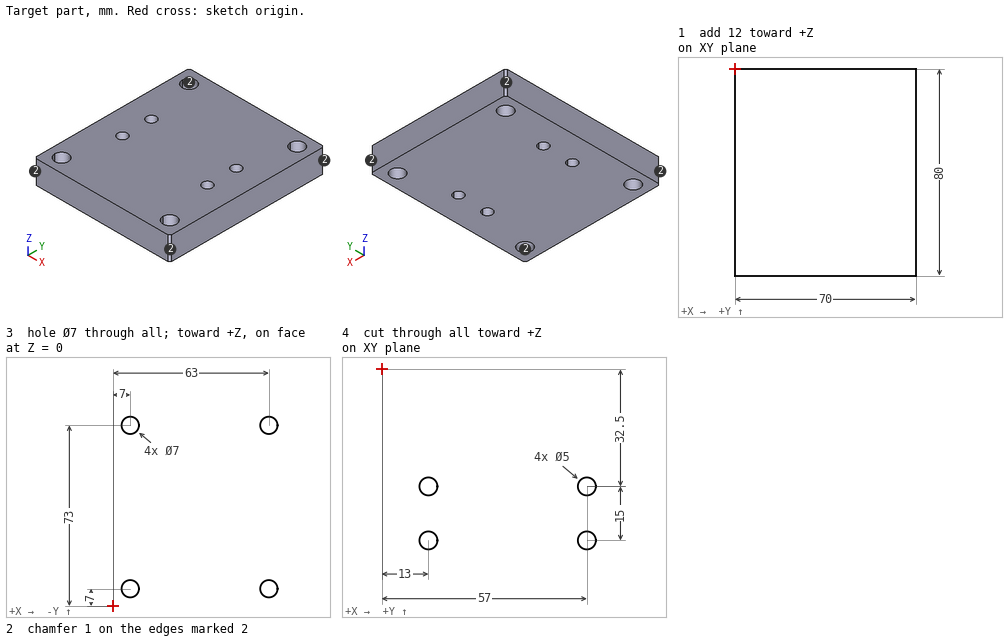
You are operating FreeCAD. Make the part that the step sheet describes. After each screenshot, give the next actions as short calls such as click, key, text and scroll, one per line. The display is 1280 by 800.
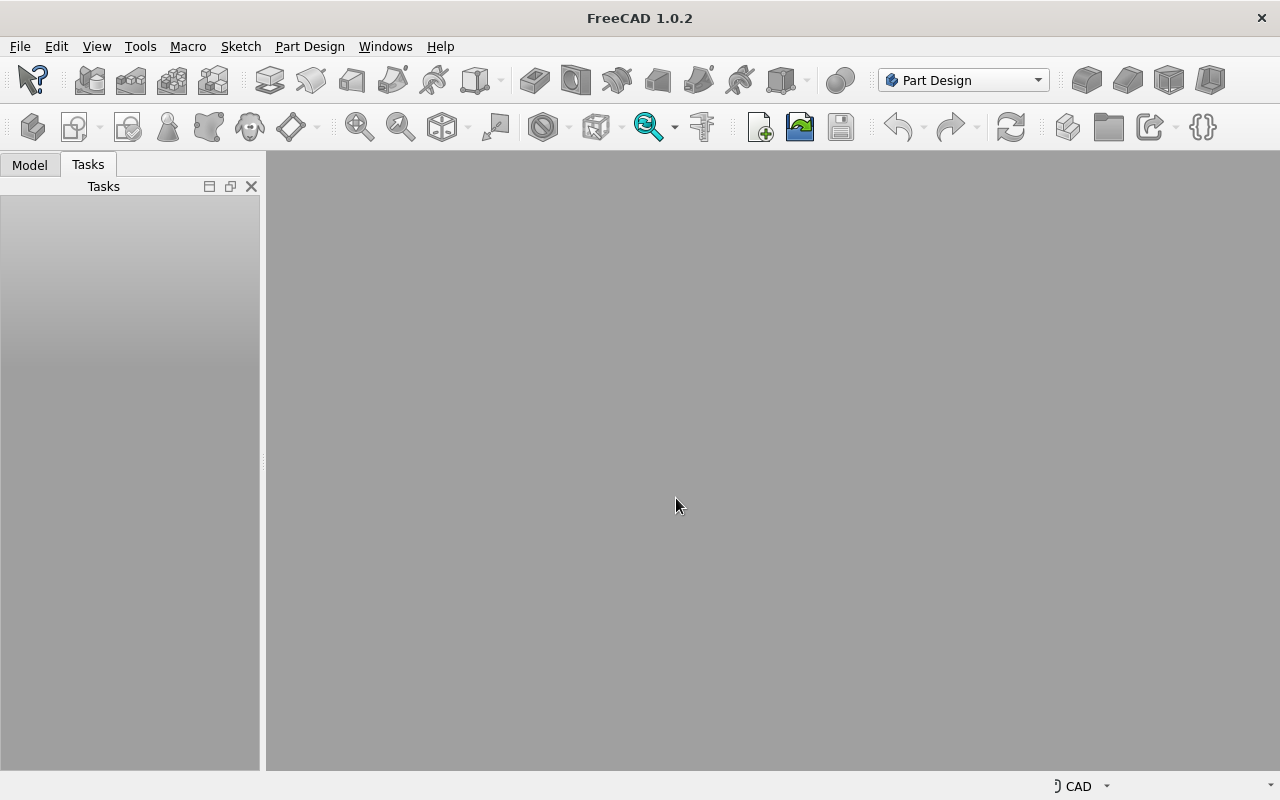
click(759, 128)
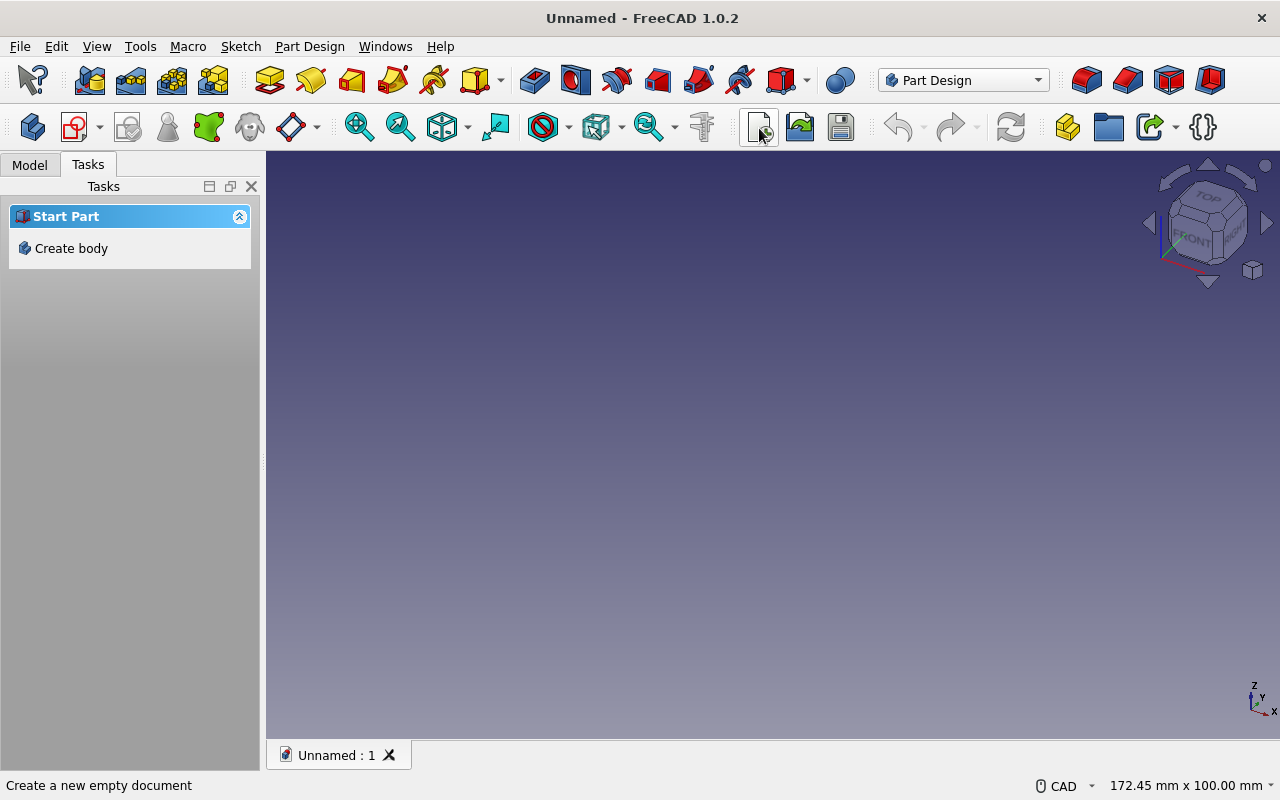
click(74, 128)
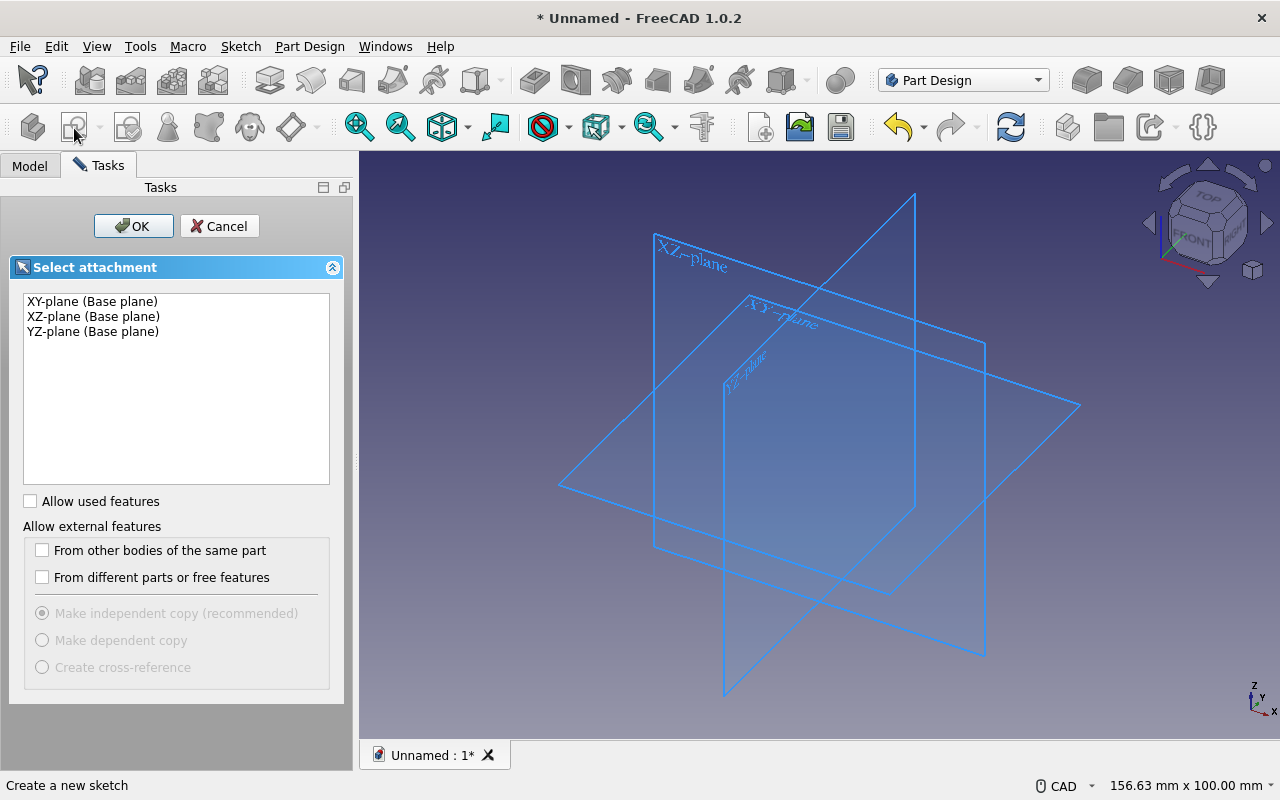
click(84, 302)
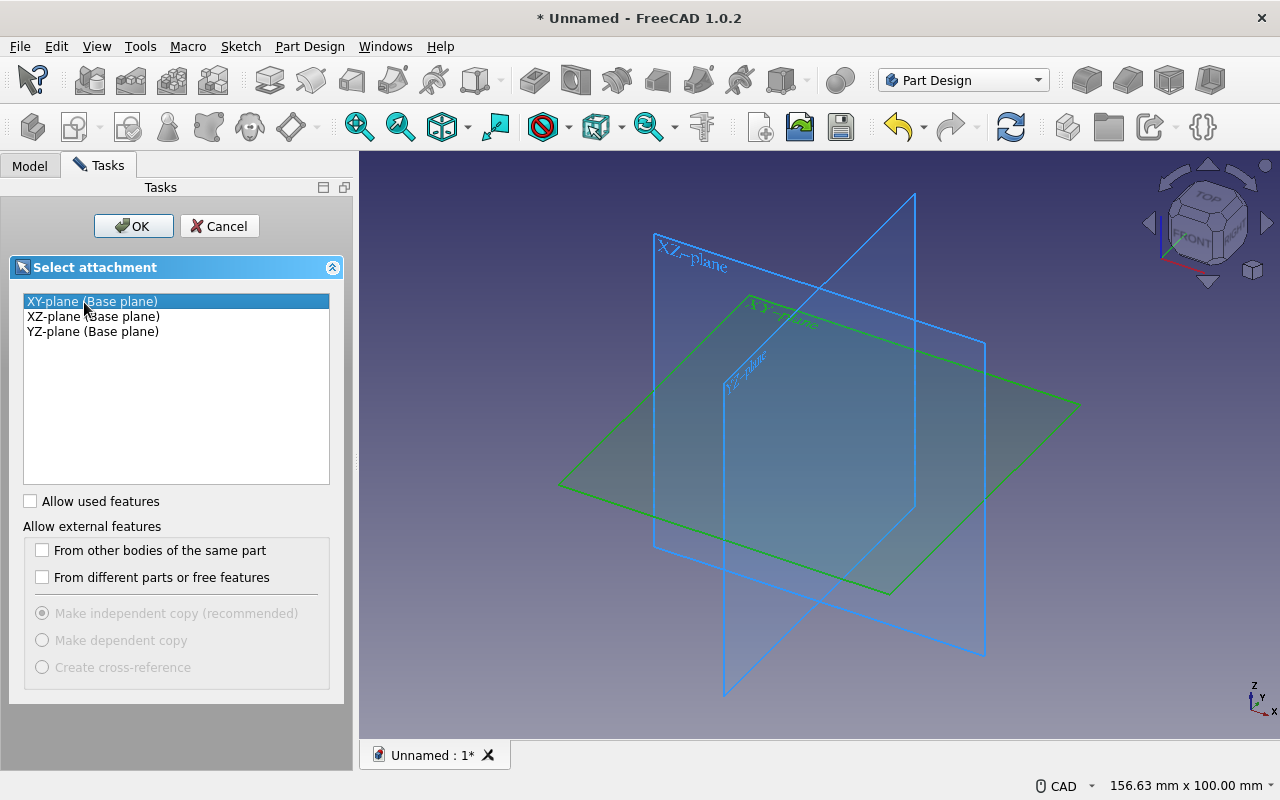
click(134, 226)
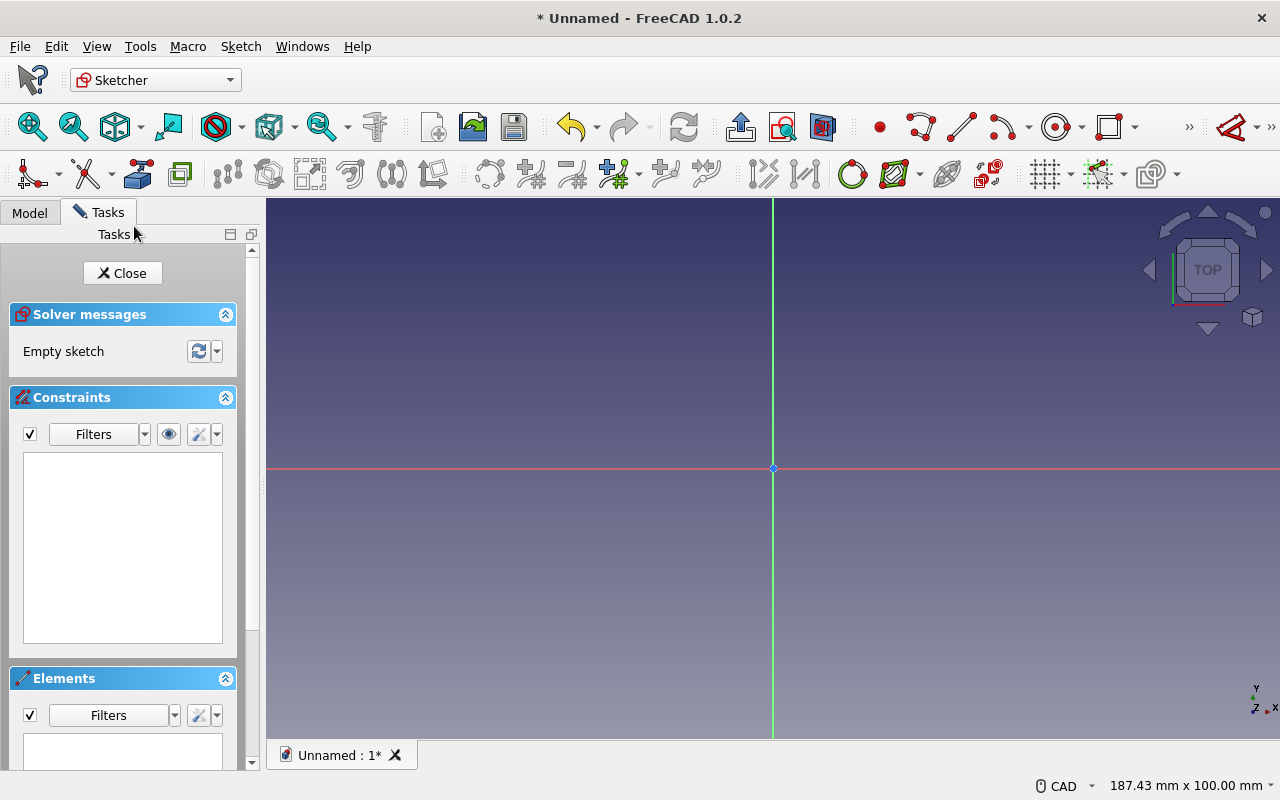
scroll(294, 226, down, 2)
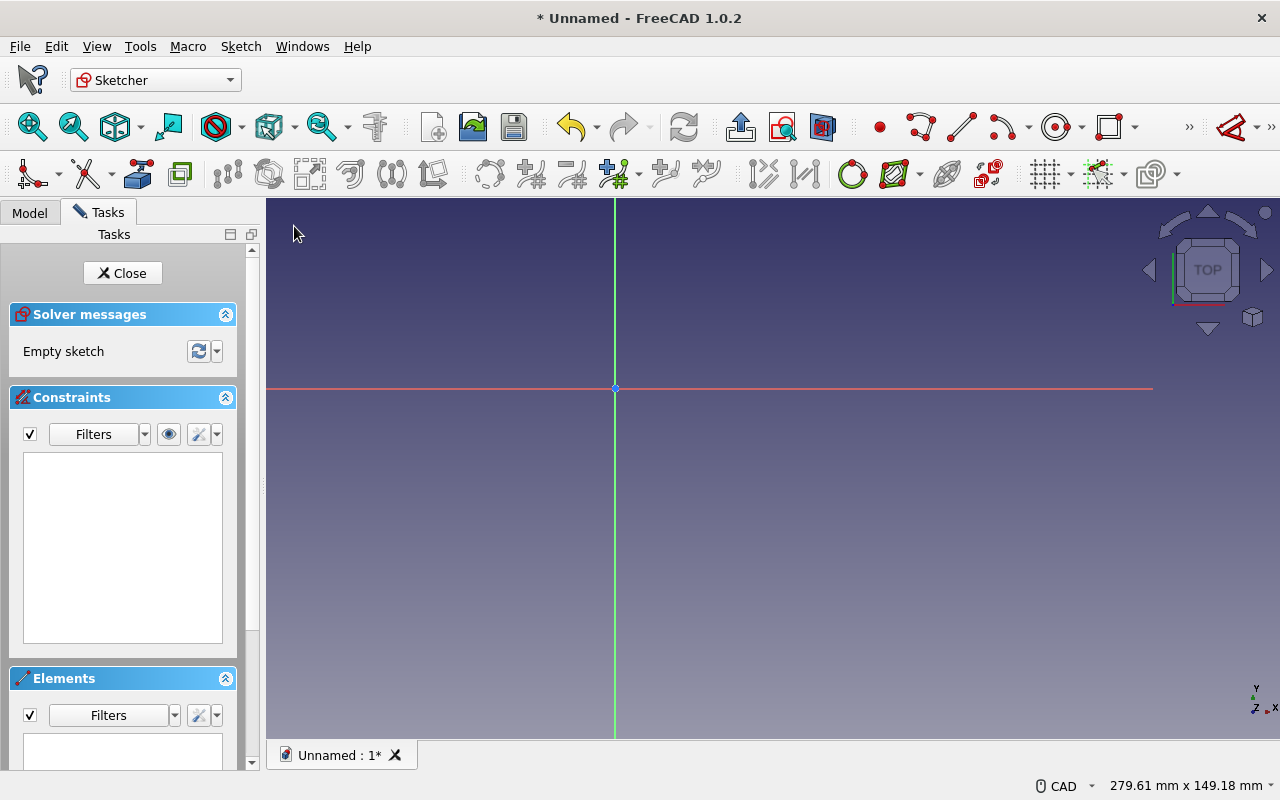
click(1108, 128)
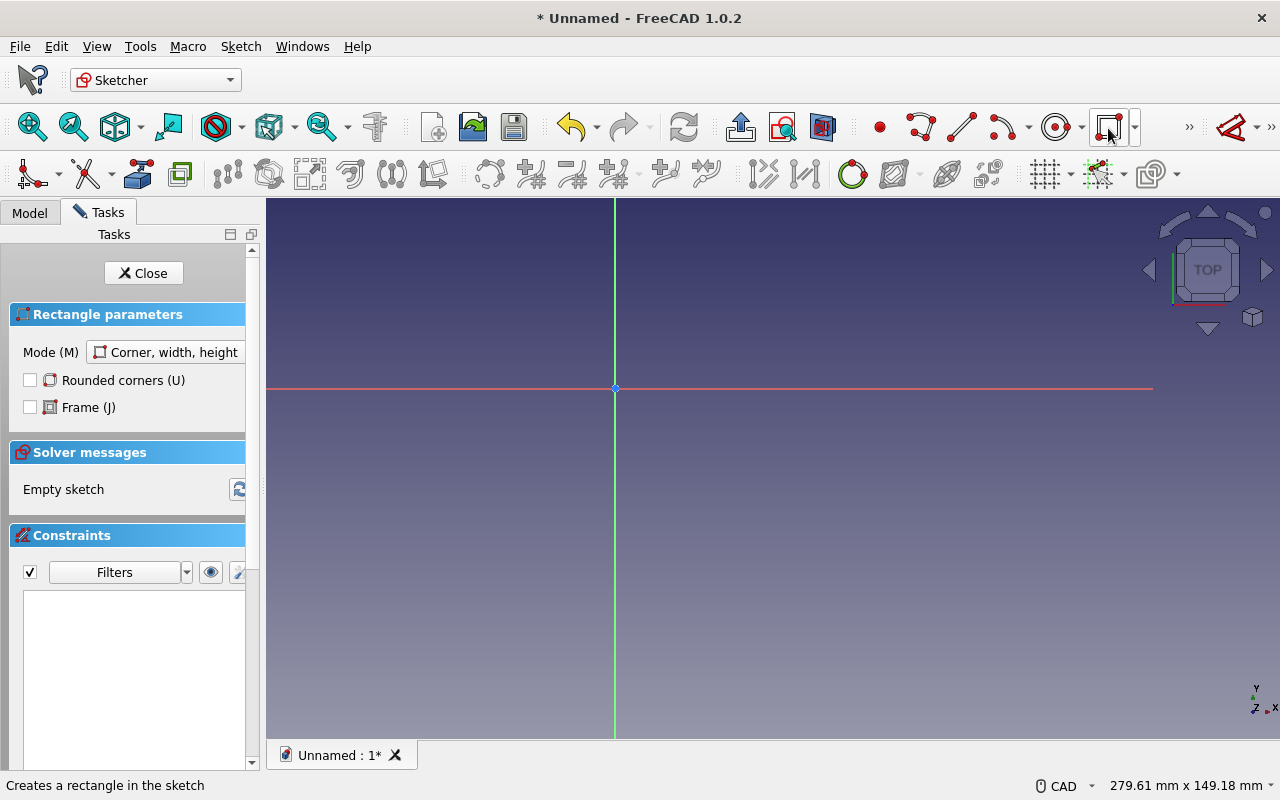
click(615, 389)
move(869, 679)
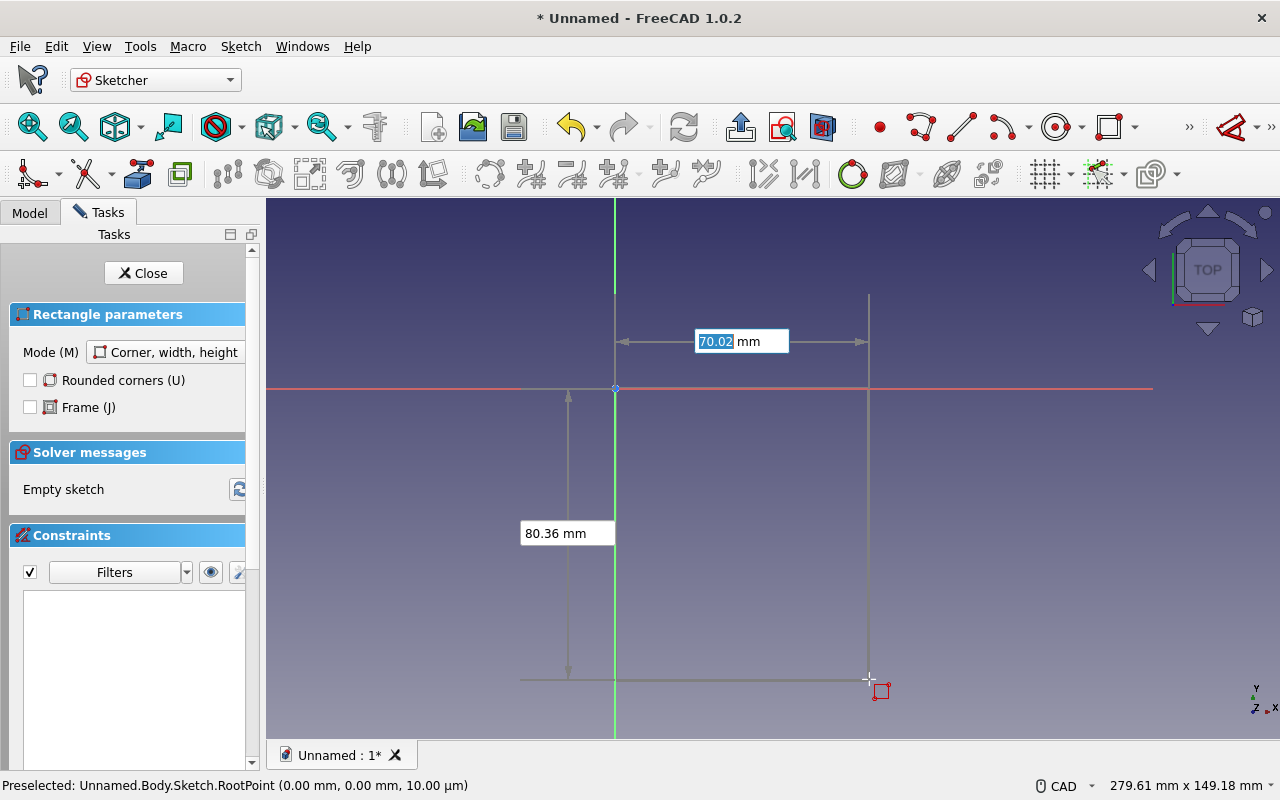
text(70)
key(Tab)
text(80)
key(Return)
key(Escape)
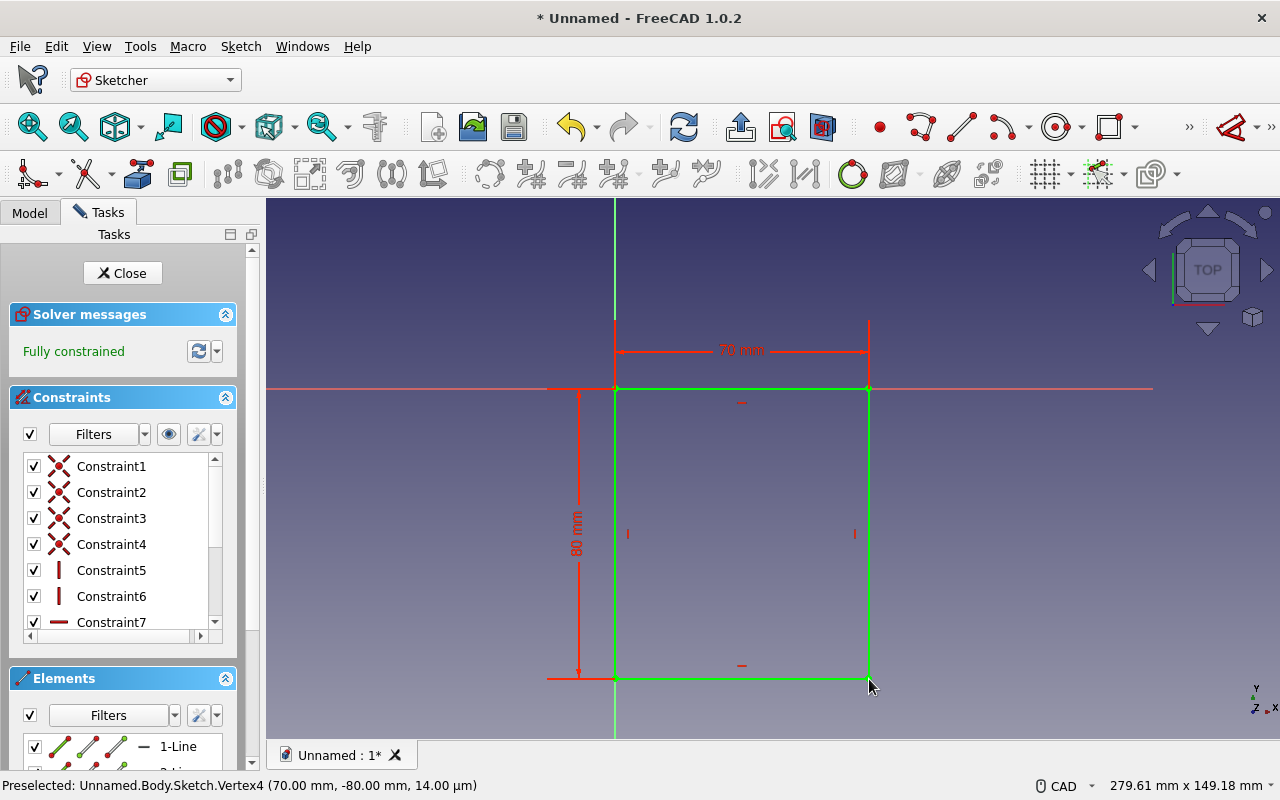
click(123, 273)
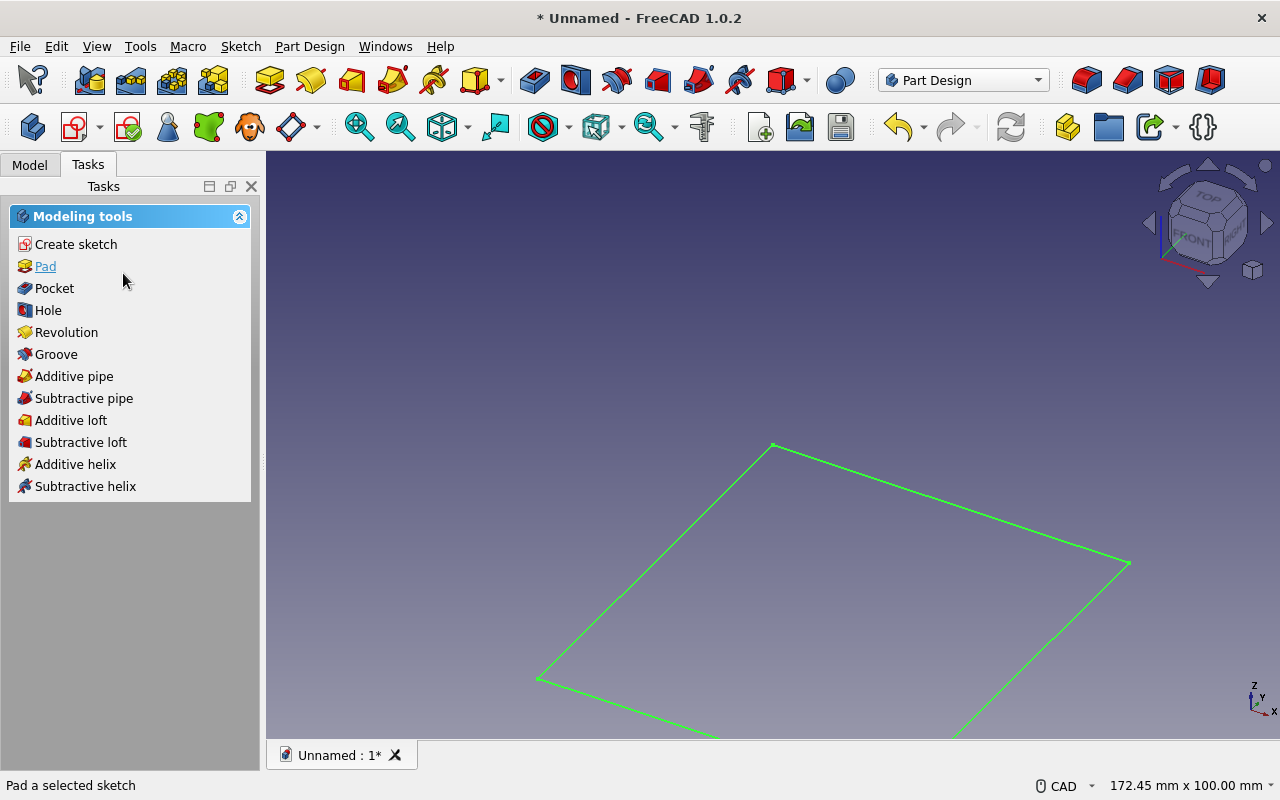
click(270, 80)